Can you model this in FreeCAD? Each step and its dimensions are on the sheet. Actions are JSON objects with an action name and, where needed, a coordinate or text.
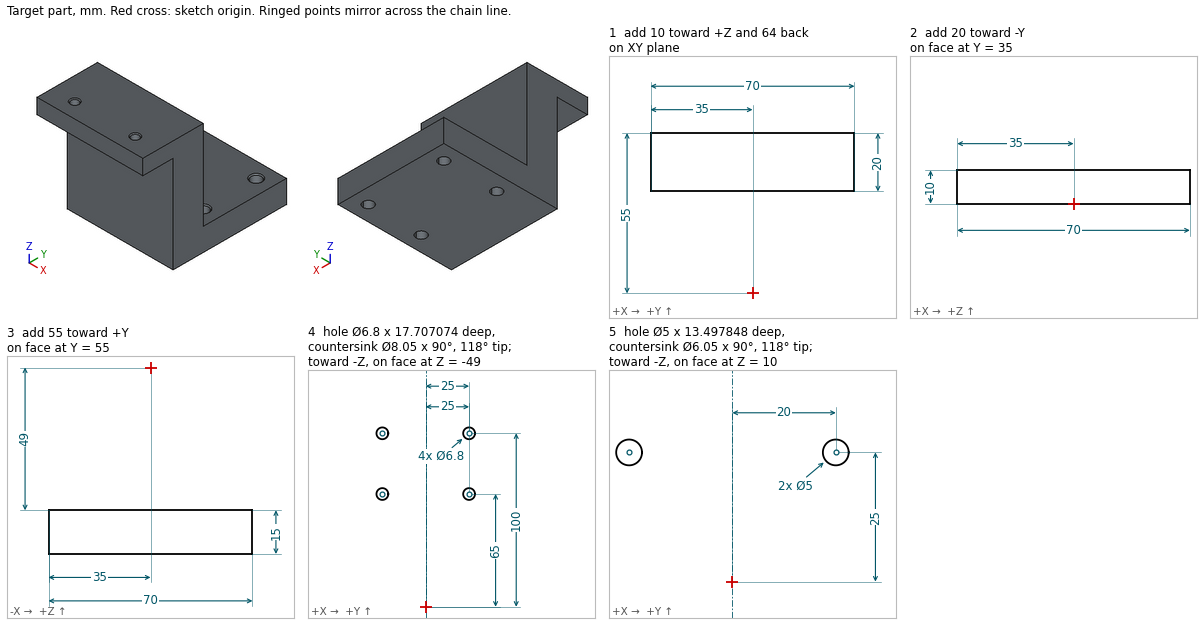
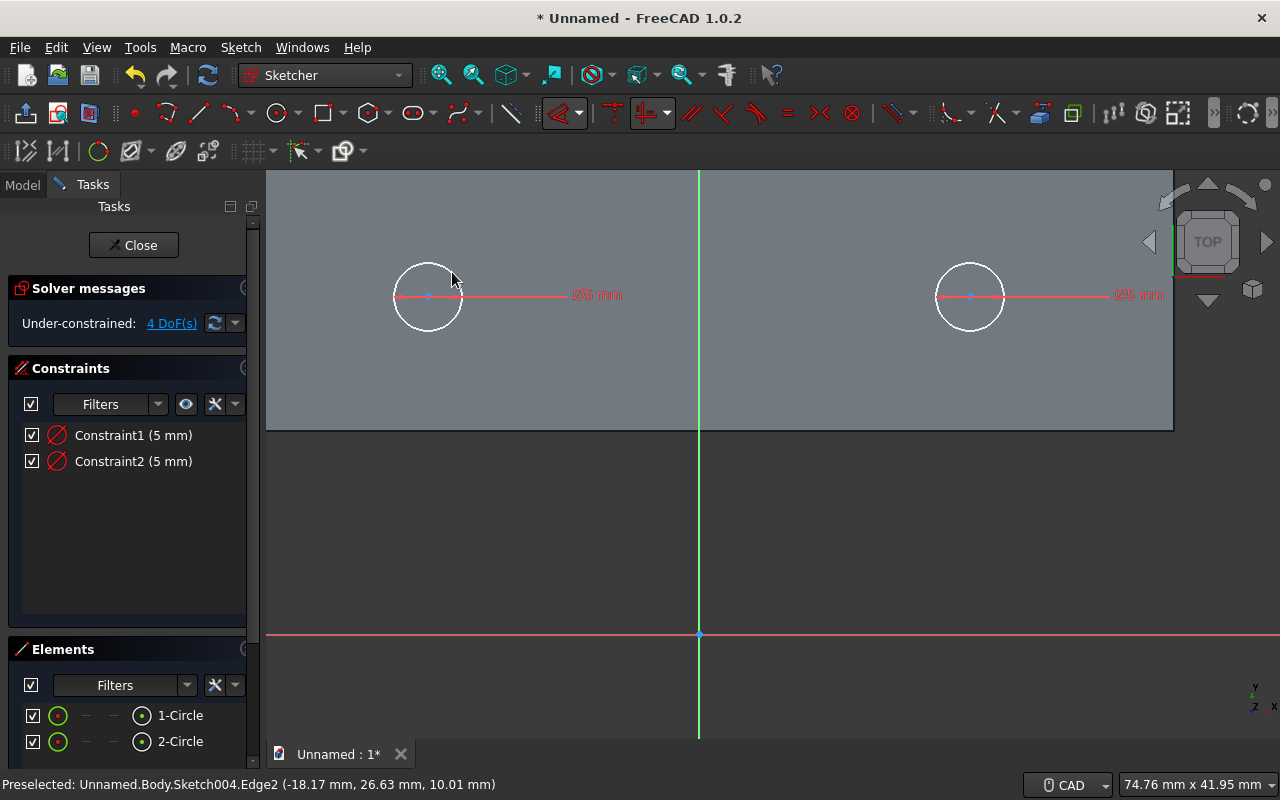
{"action": "left_click", "coordinate": [970, 297]}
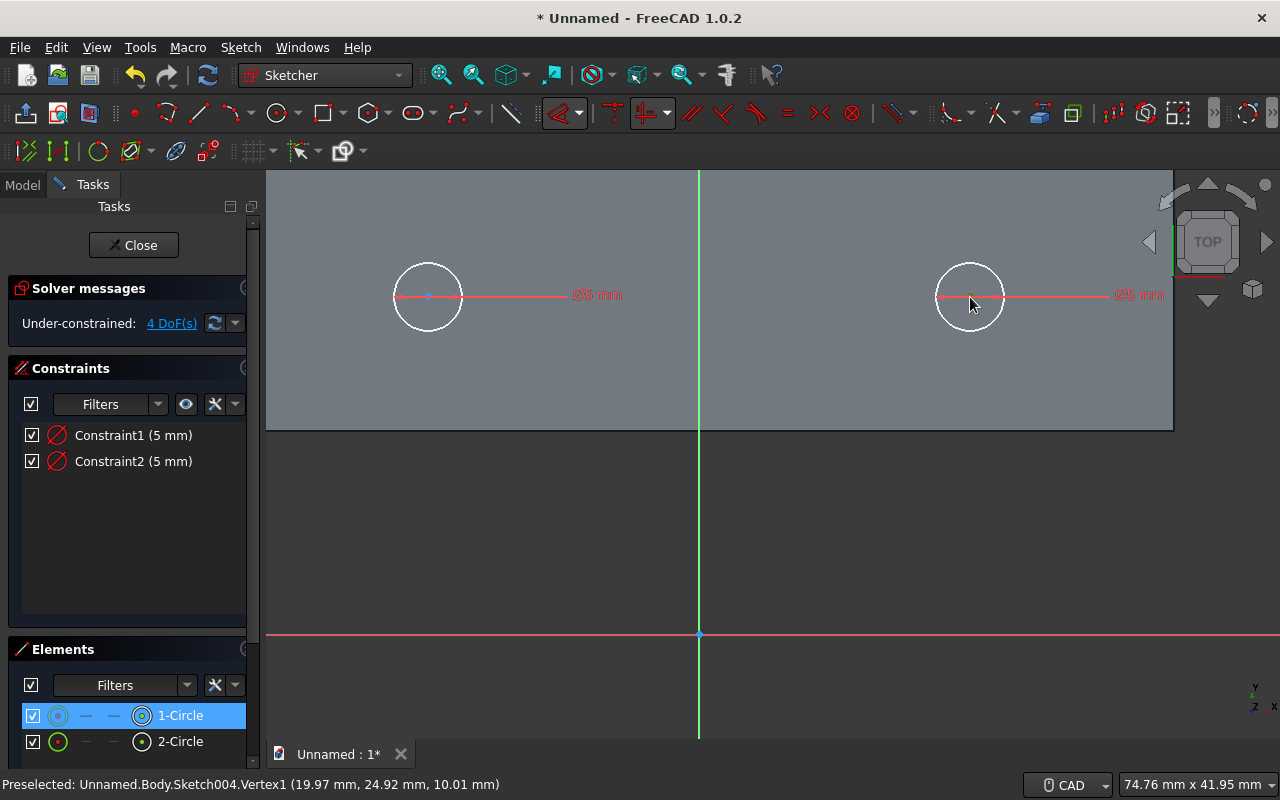
{"action": "left_click", "coordinate": [428, 297]}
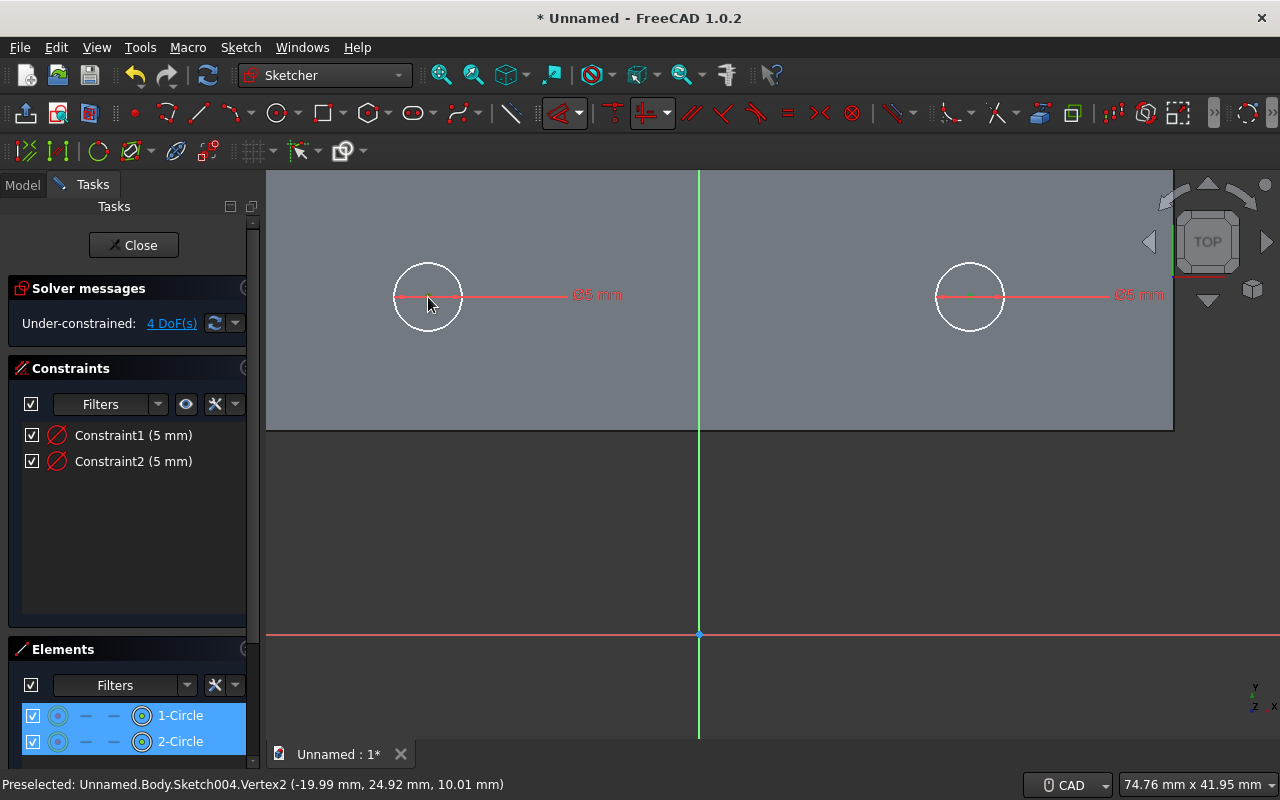
{"action": "left_click", "coordinate": [699, 674]}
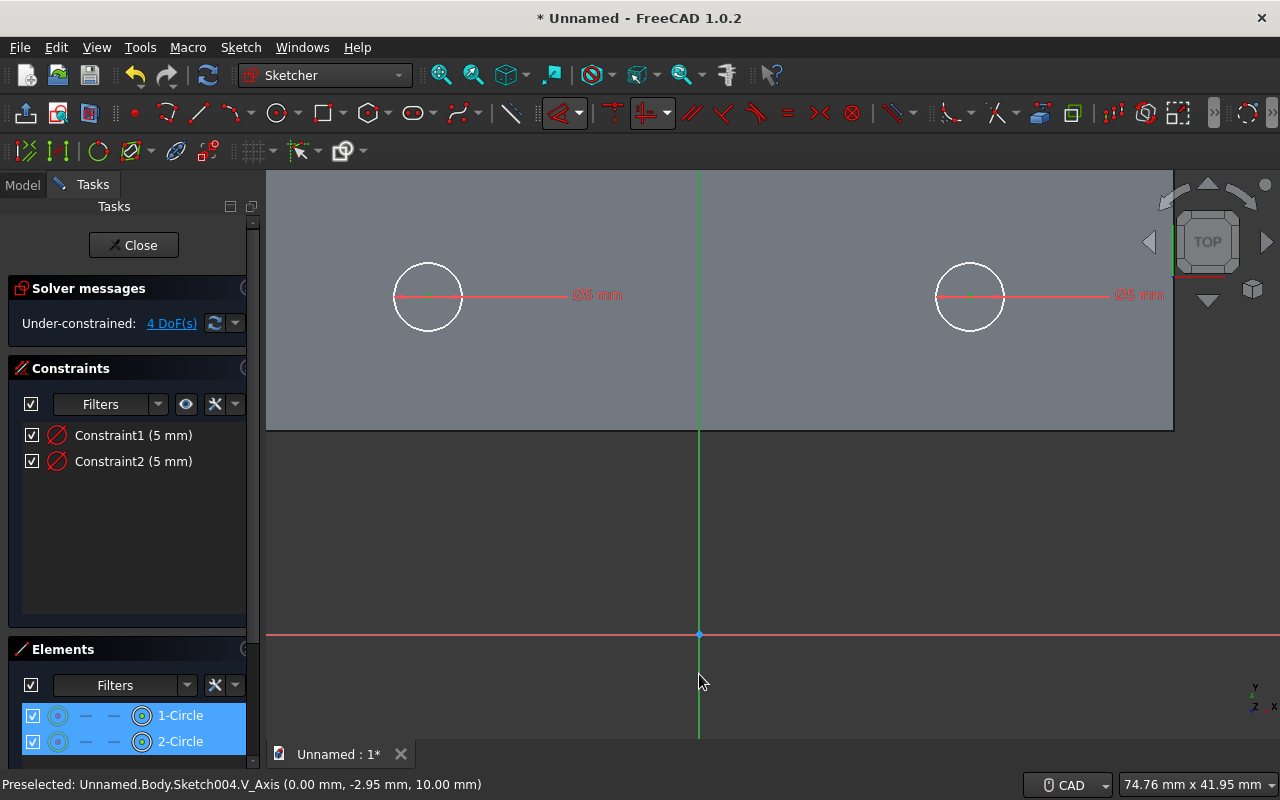
{"action": "key", "text": "s"}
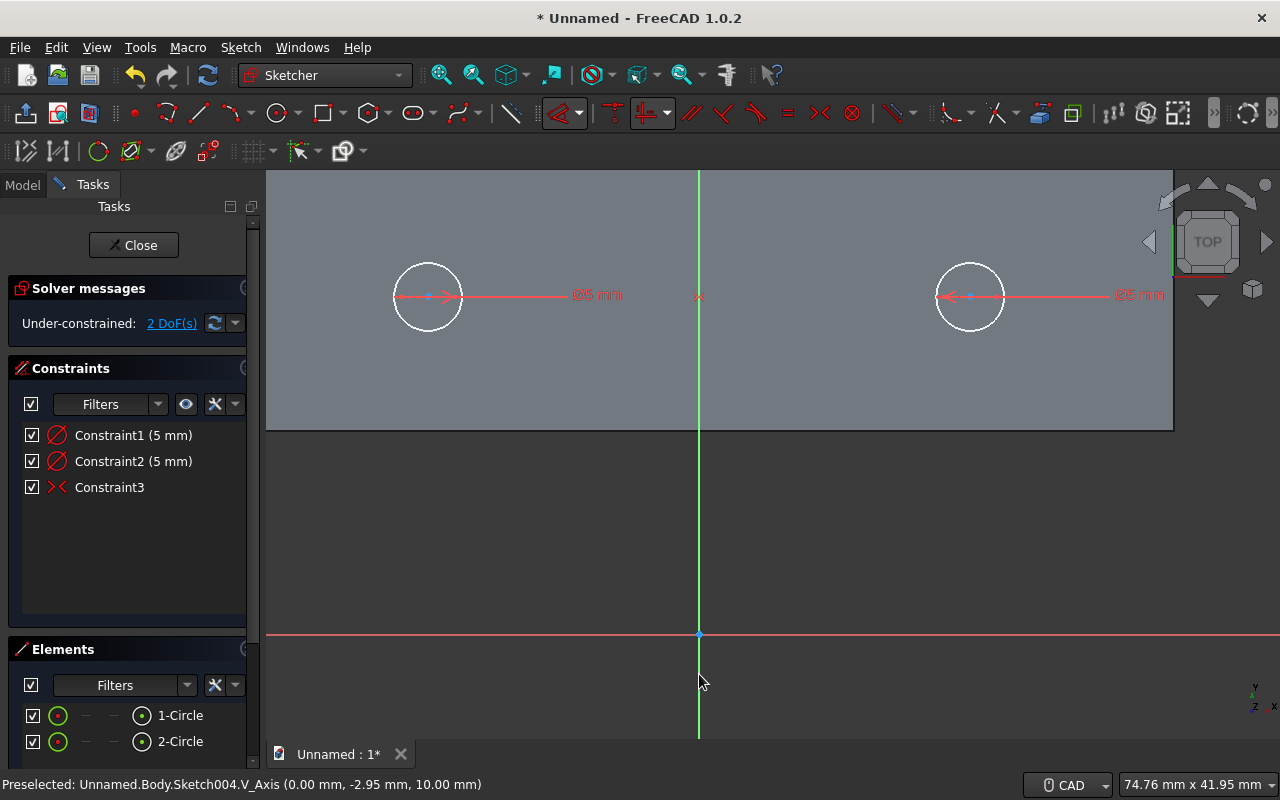
{"action": "left_click", "coordinate": [970, 297]}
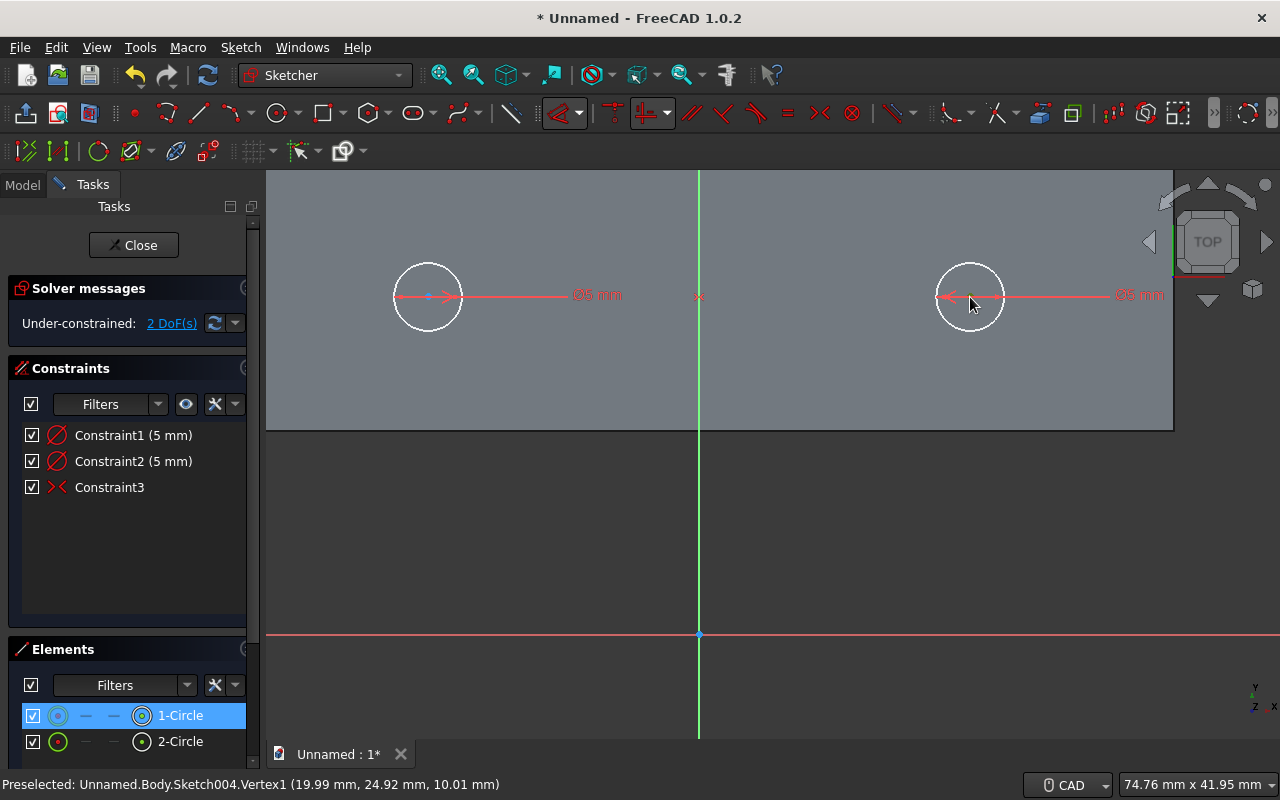
{"action": "key", "text": "l"}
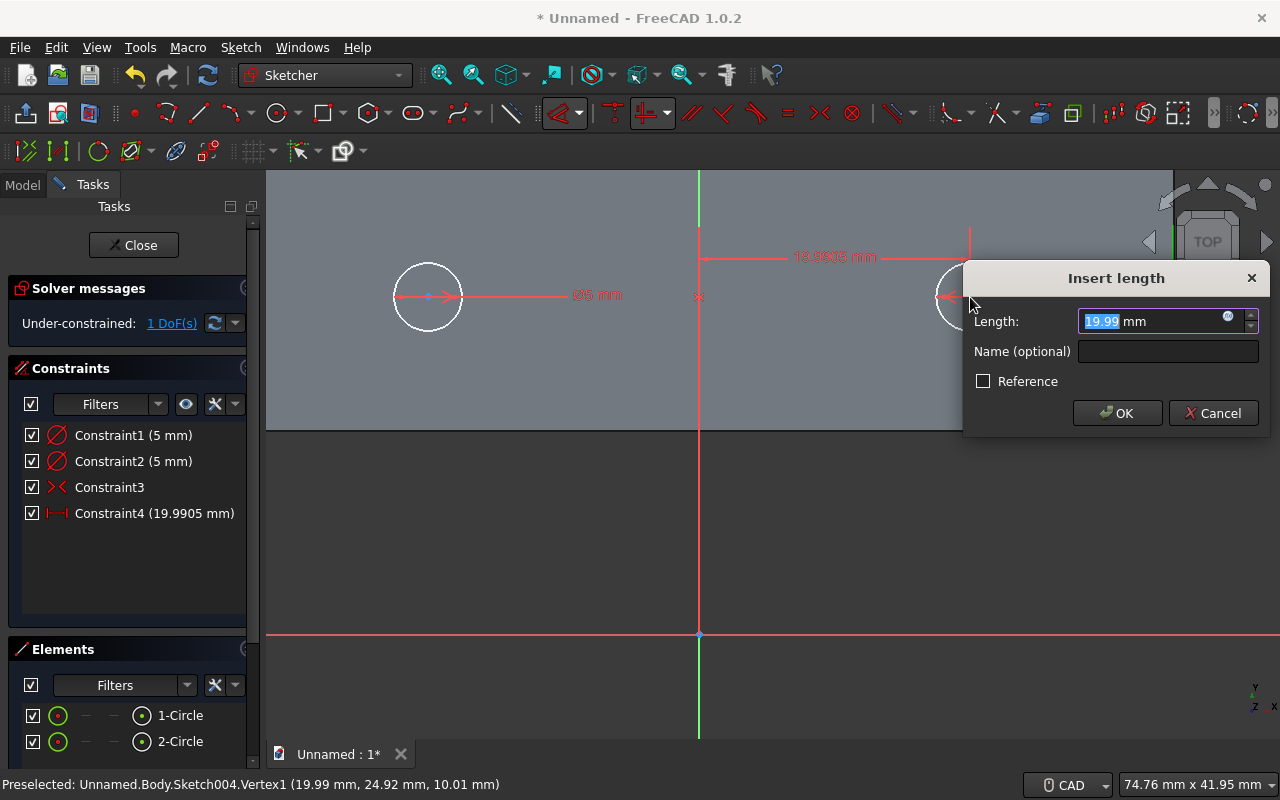
{"action": "type", "text": "20"}
{"action": "key", "text": "Return"}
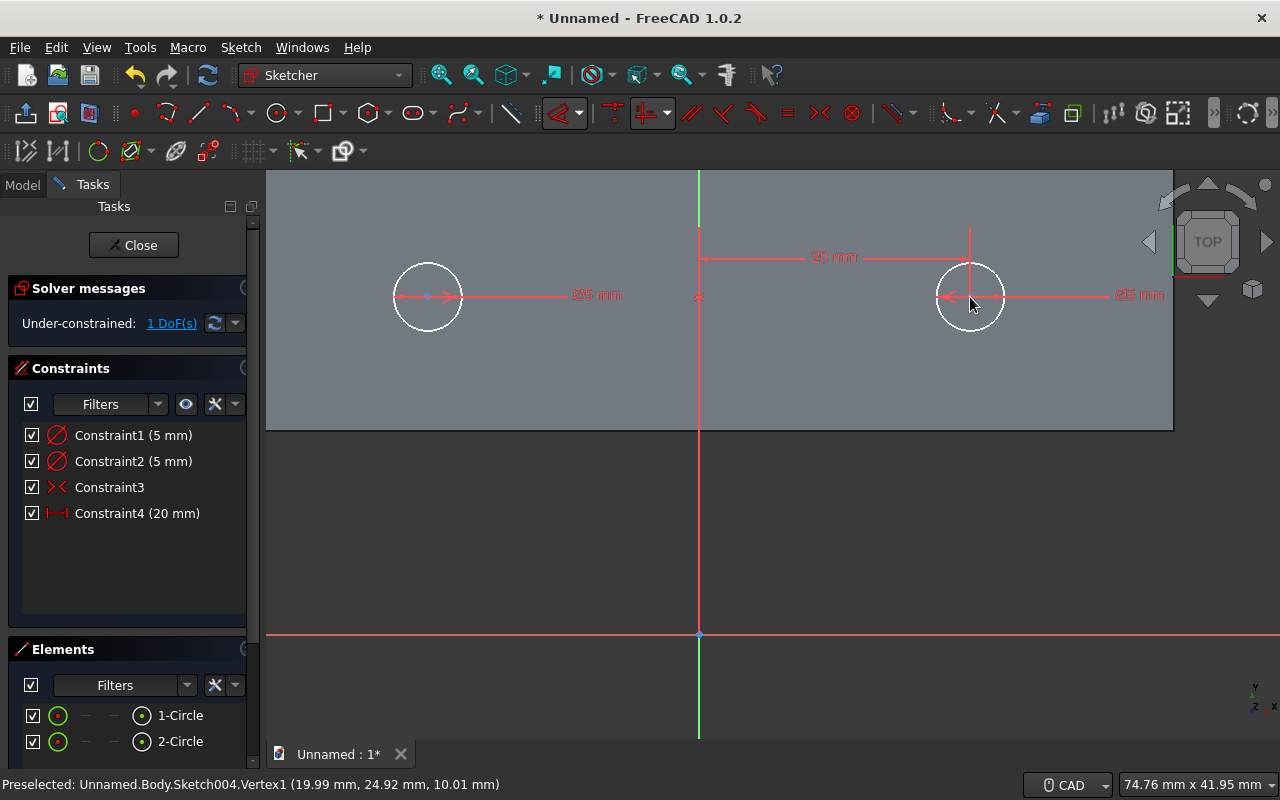
{"action": "left_click", "coordinate": [970, 297]}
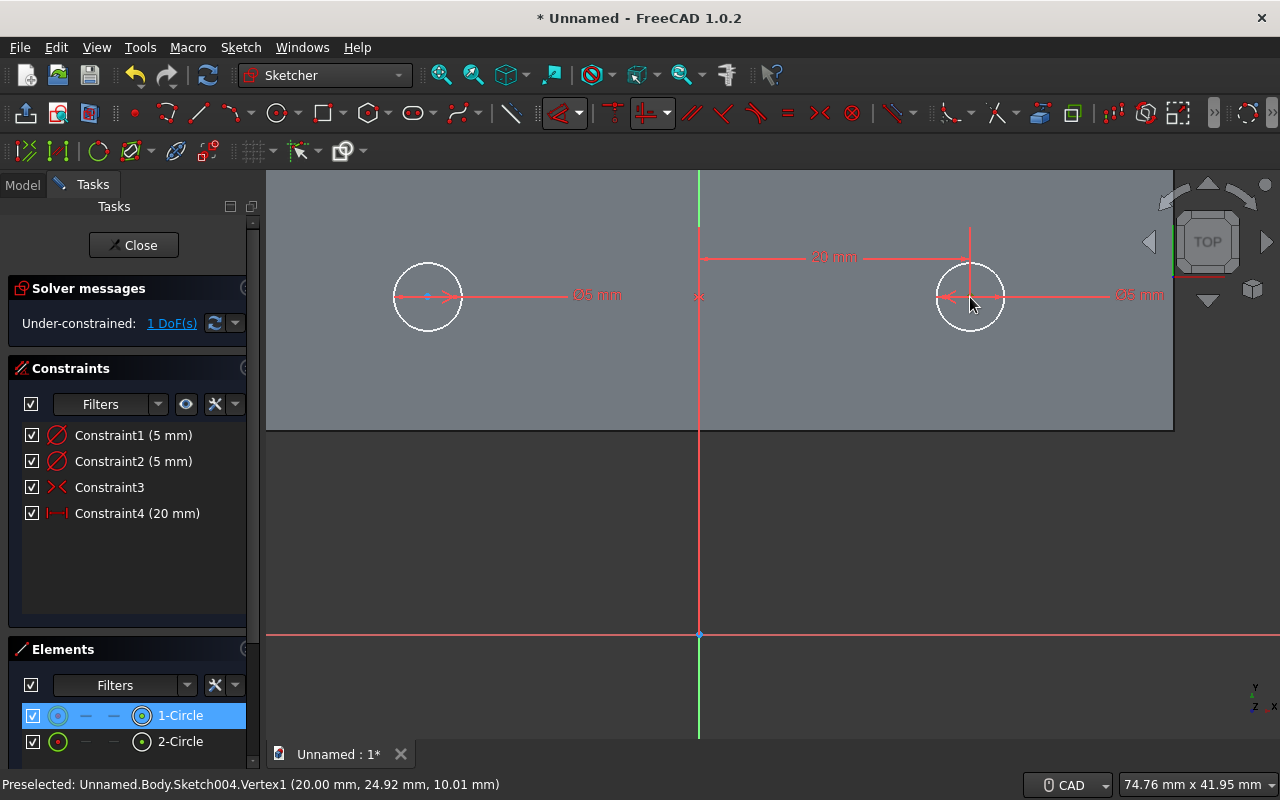
{"action": "key", "text": "i"}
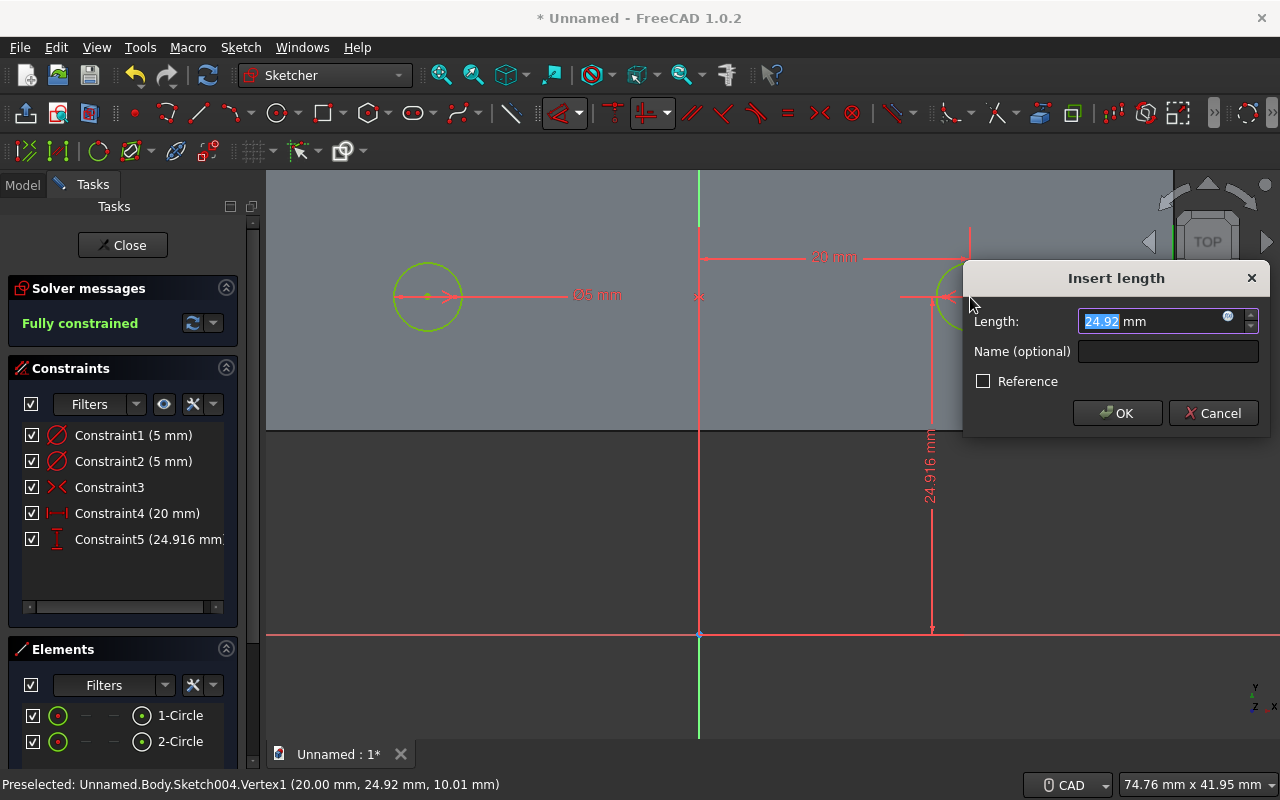
{"action": "type", "text": "25"}
{"action": "key", "text": "Return"}